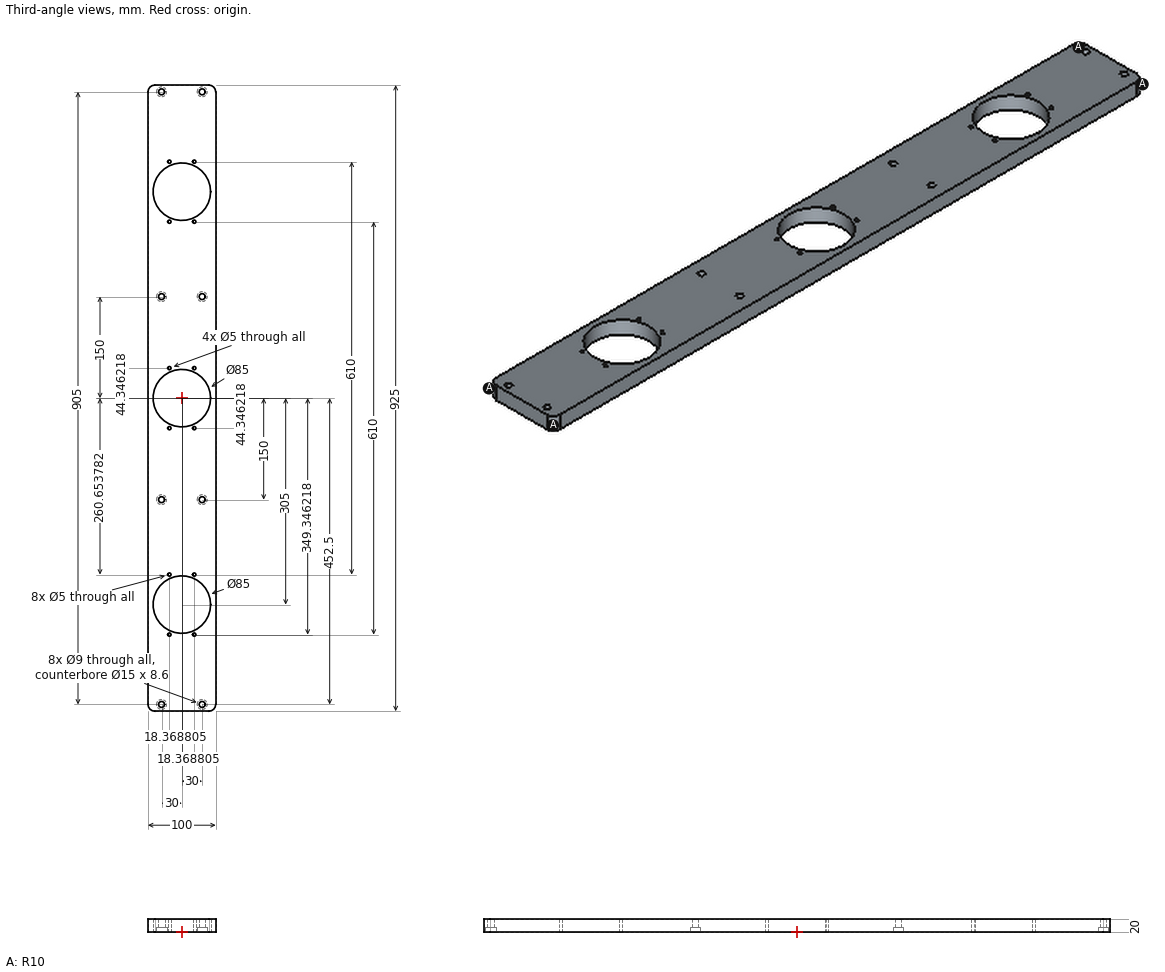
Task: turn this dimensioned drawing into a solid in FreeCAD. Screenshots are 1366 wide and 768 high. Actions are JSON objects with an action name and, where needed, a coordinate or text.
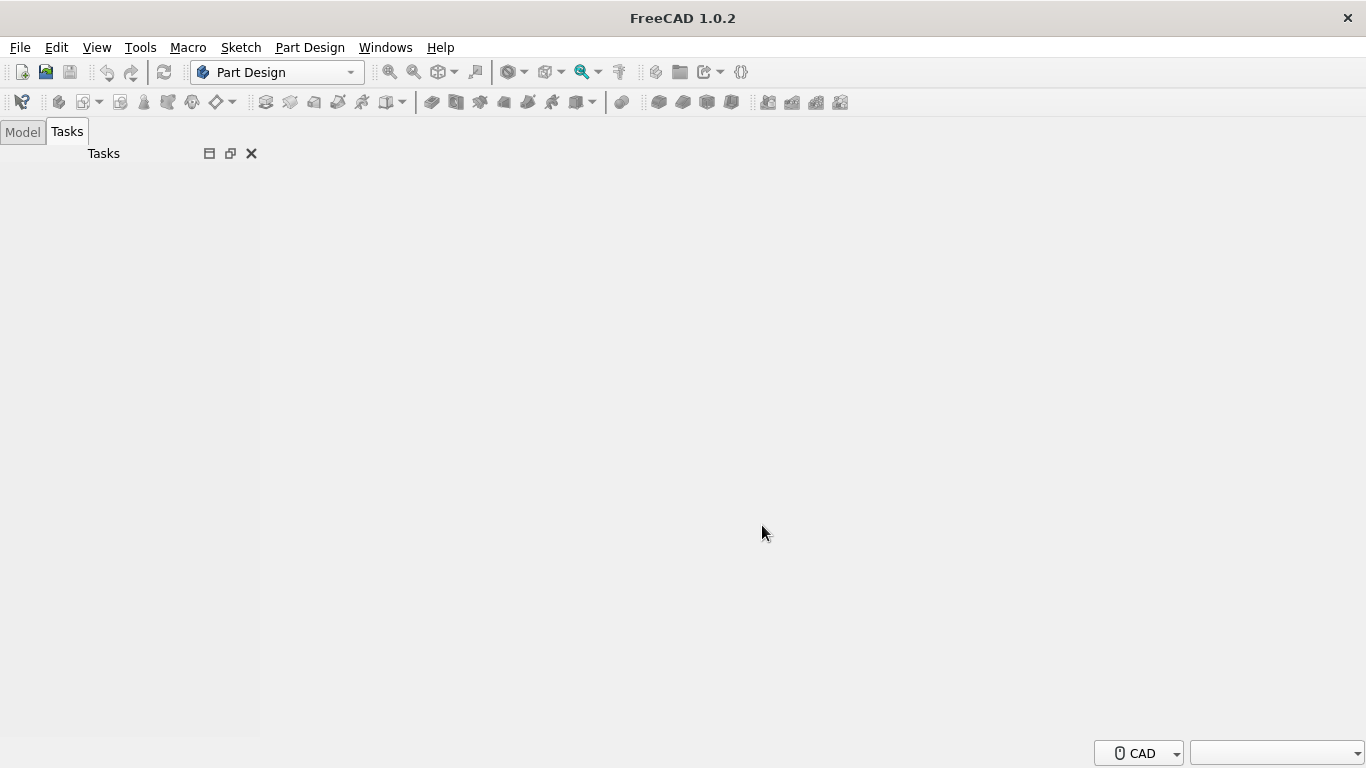
{"action": "key", "text": "ctrl+n"}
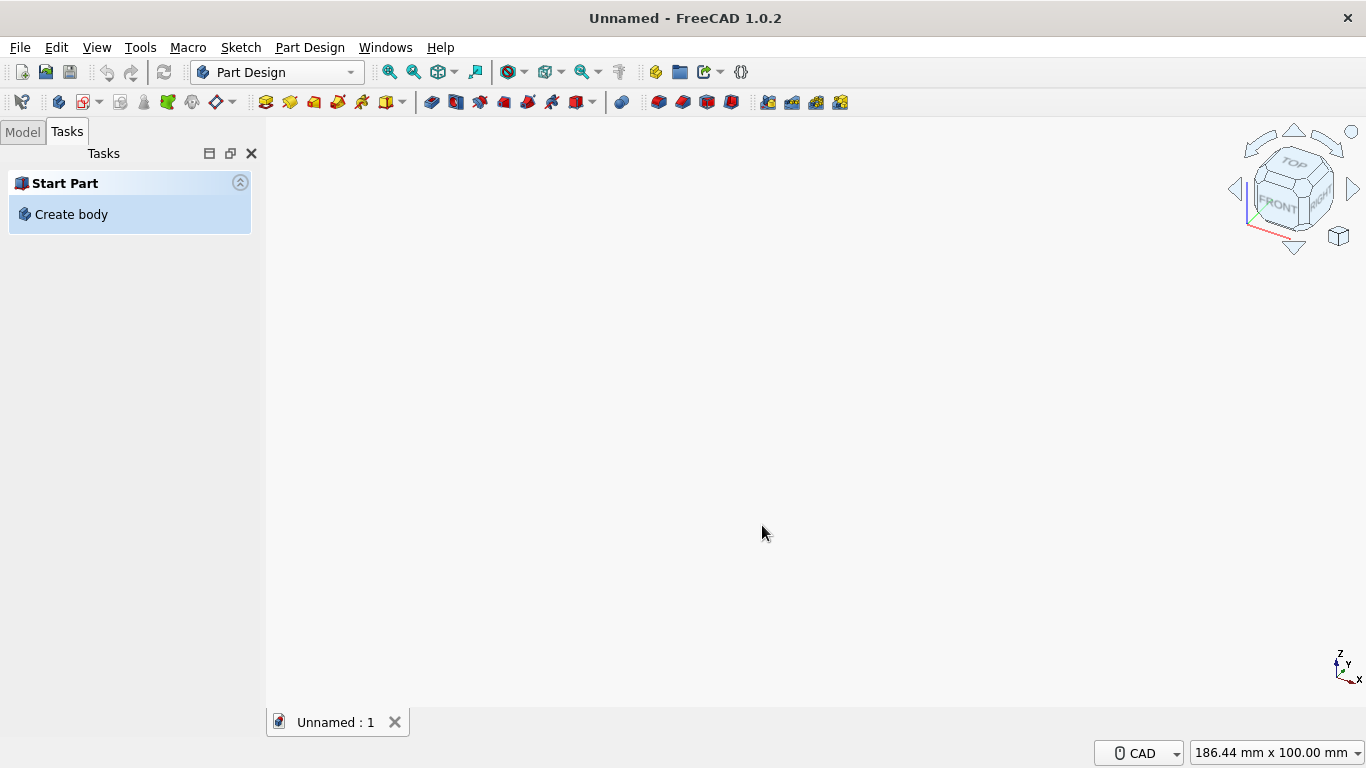
{"action": "left_click", "coordinate": [84, 102]}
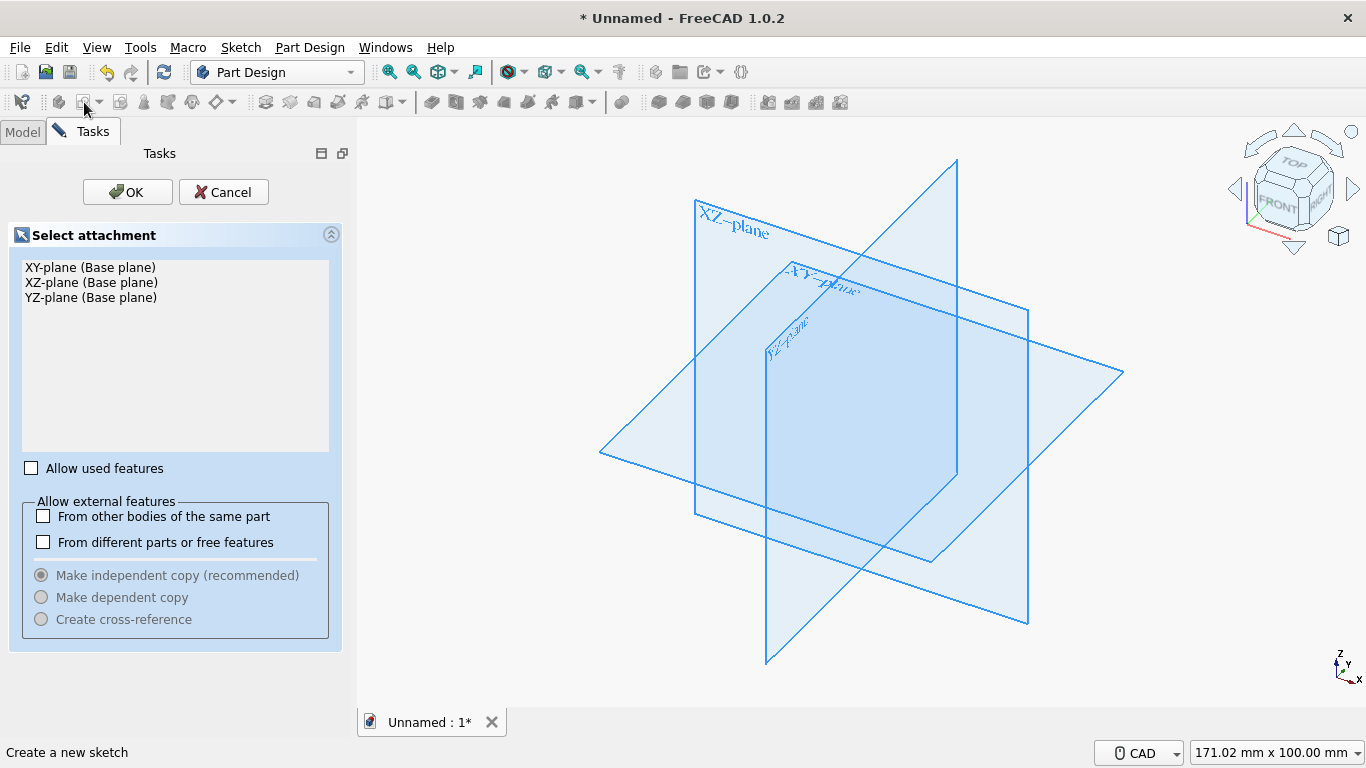
{"action": "left_click", "coordinate": [82, 268]}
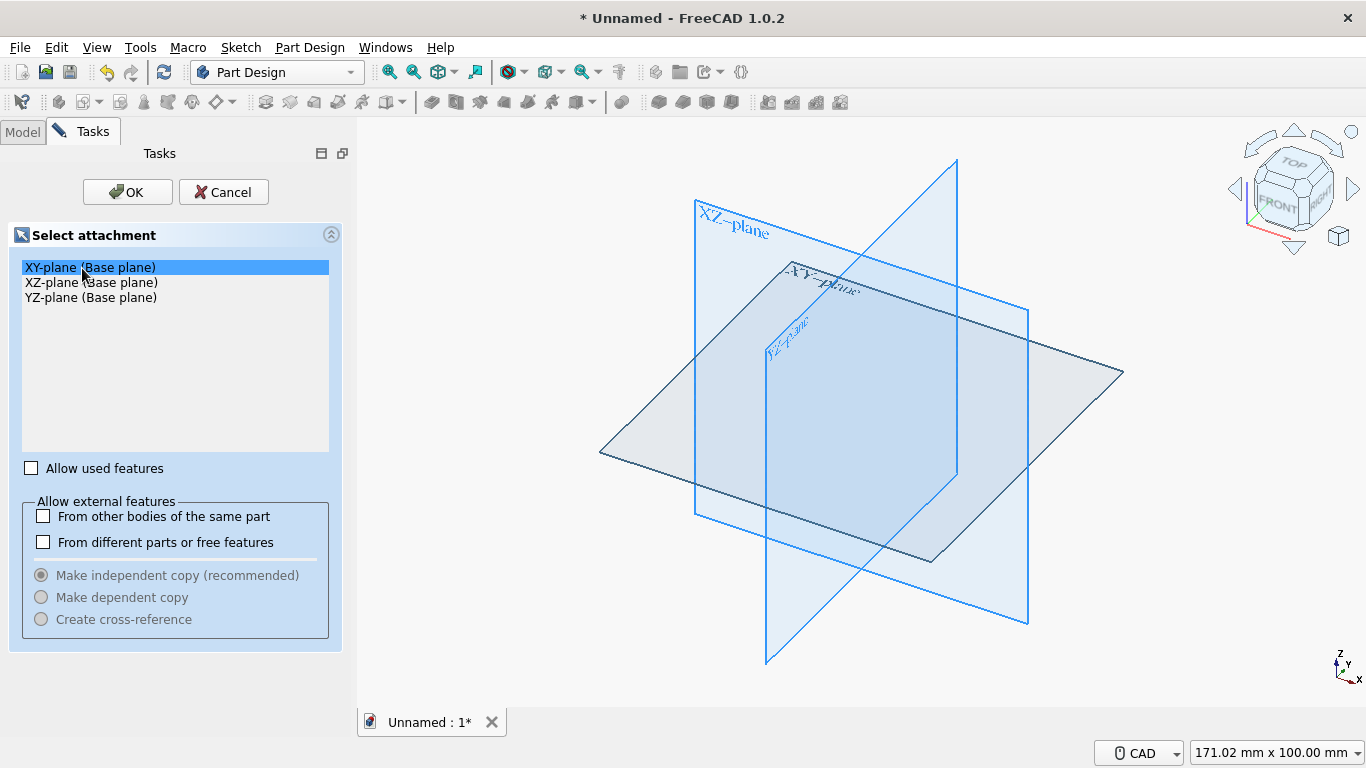
{"action": "left_click", "coordinate": [128, 192]}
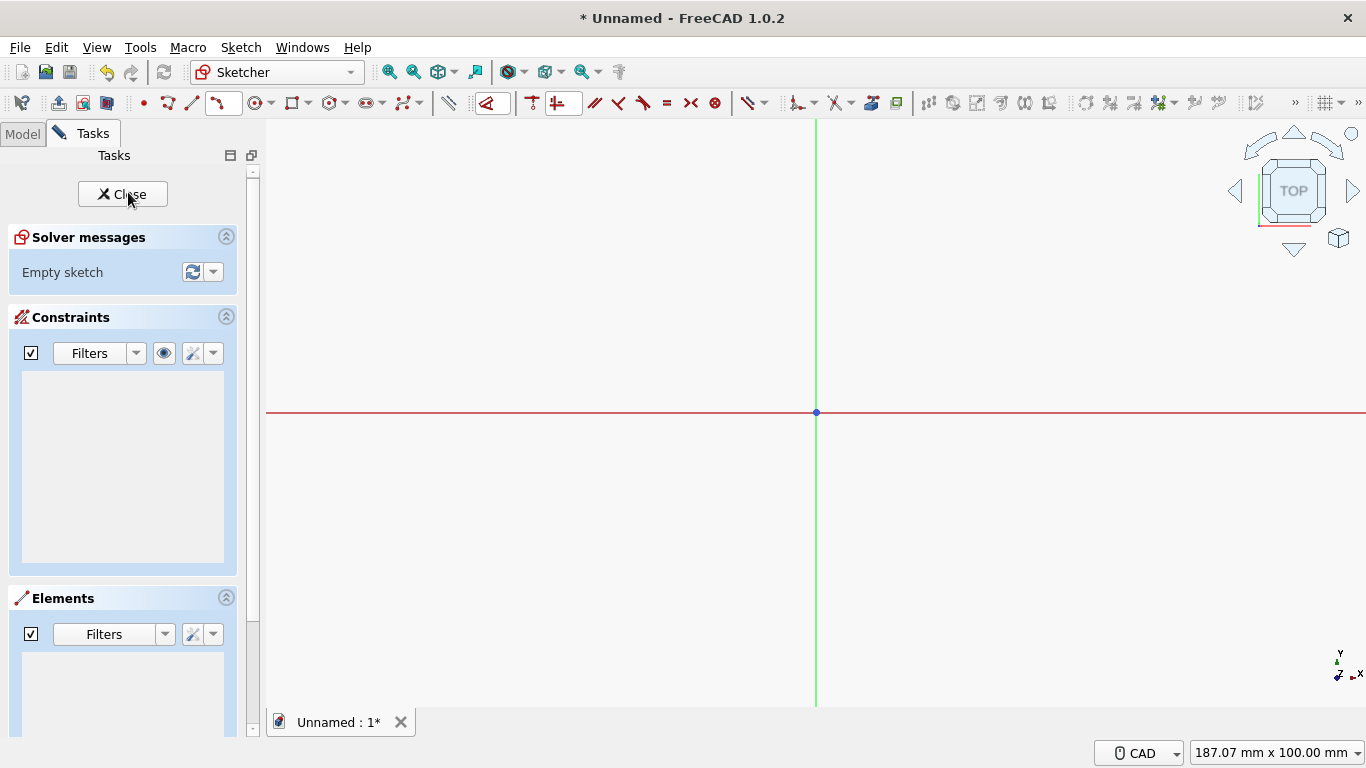
{"action": "scroll", "coordinate": [742, 413], "scroll_direction": "down", "scroll_amount": 13}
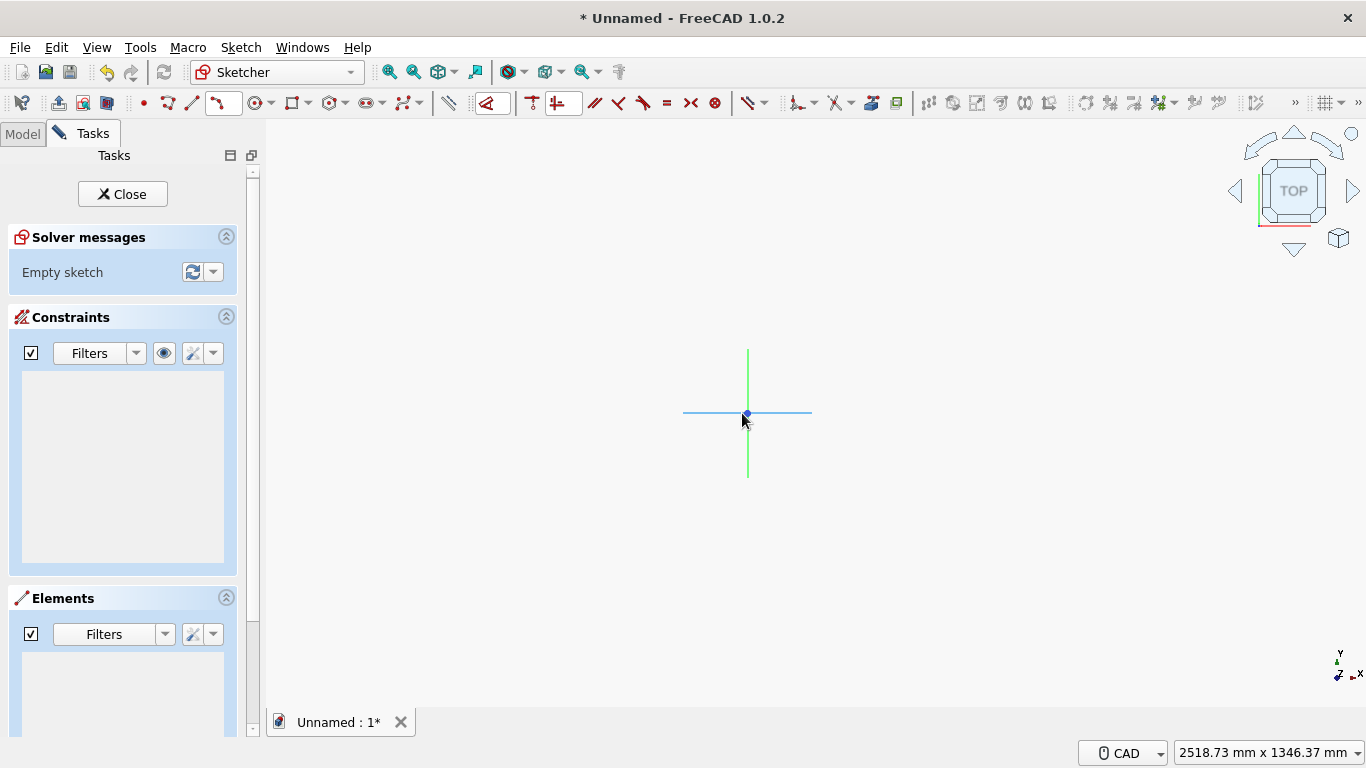
{"action": "key", "text": "g v"}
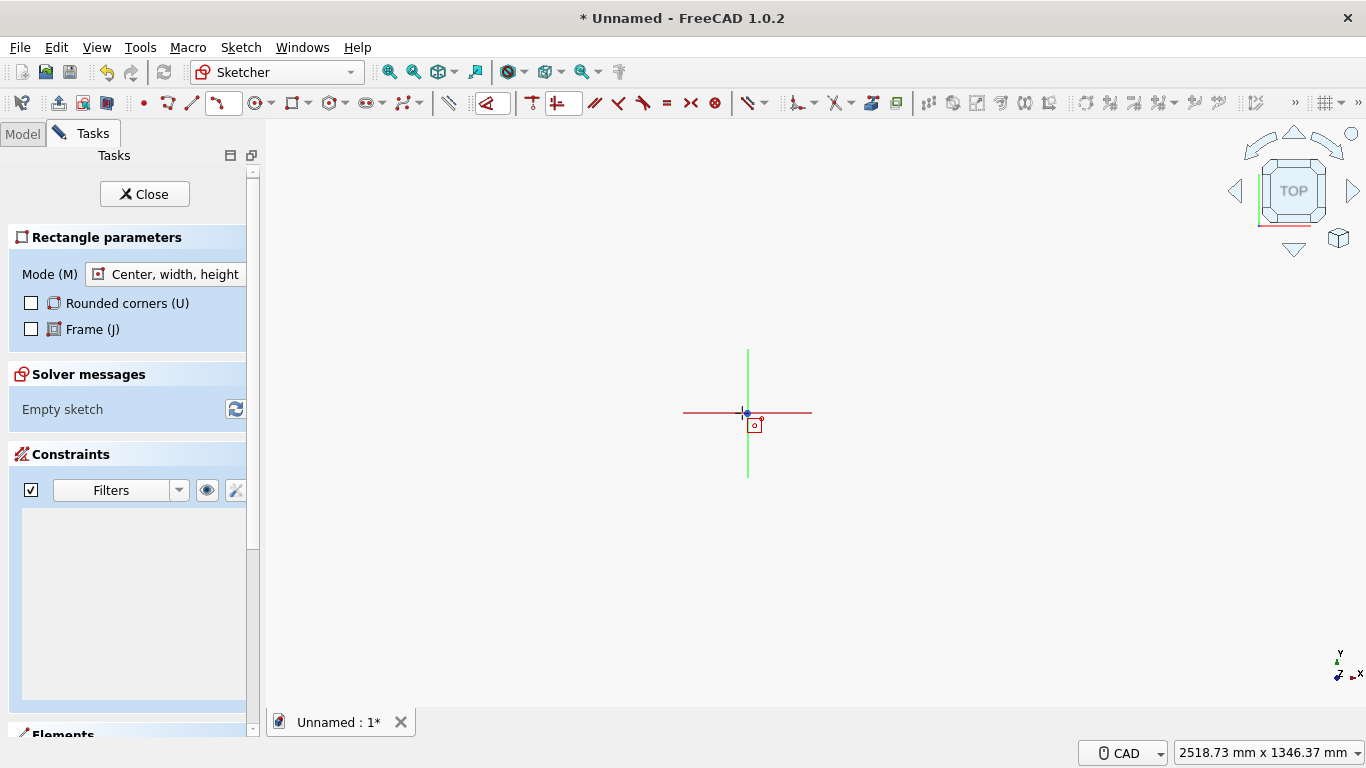
{"action": "left_click", "coordinate": [748, 413]}
{"action": "left_click", "coordinate": [770, 211]}
{"action": "key", "text": "Escape"}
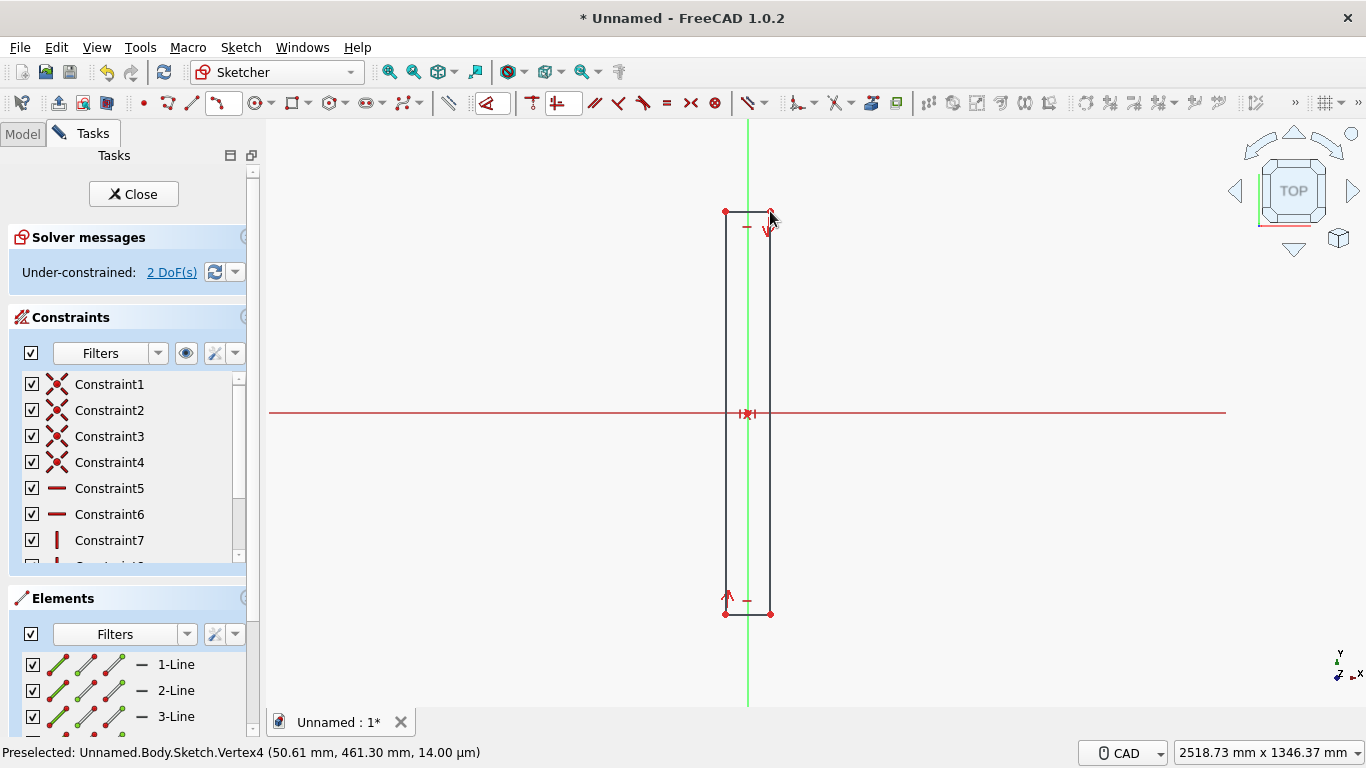
{"action": "key", "text": "d"}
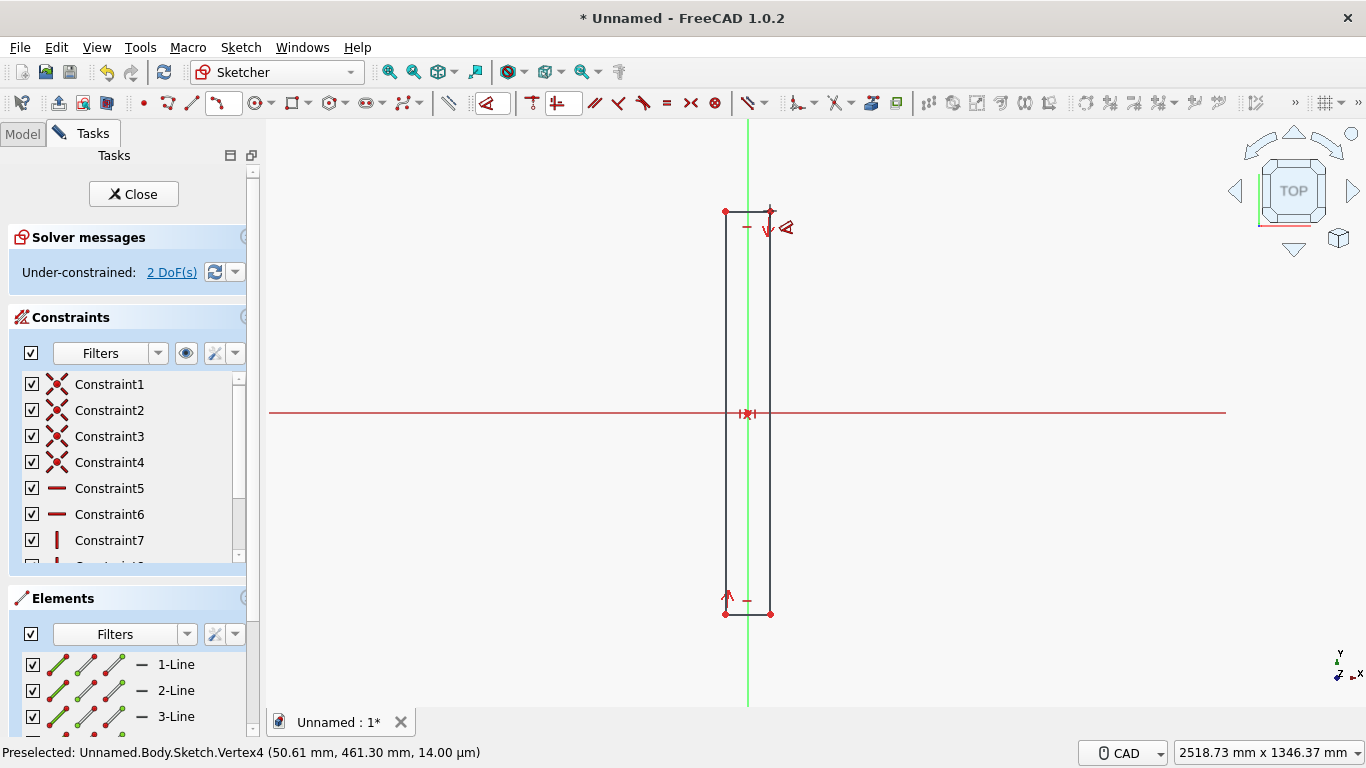
{"action": "left_click", "coordinate": [748, 615]}
{"action": "left_click", "coordinate": [732, 649]}